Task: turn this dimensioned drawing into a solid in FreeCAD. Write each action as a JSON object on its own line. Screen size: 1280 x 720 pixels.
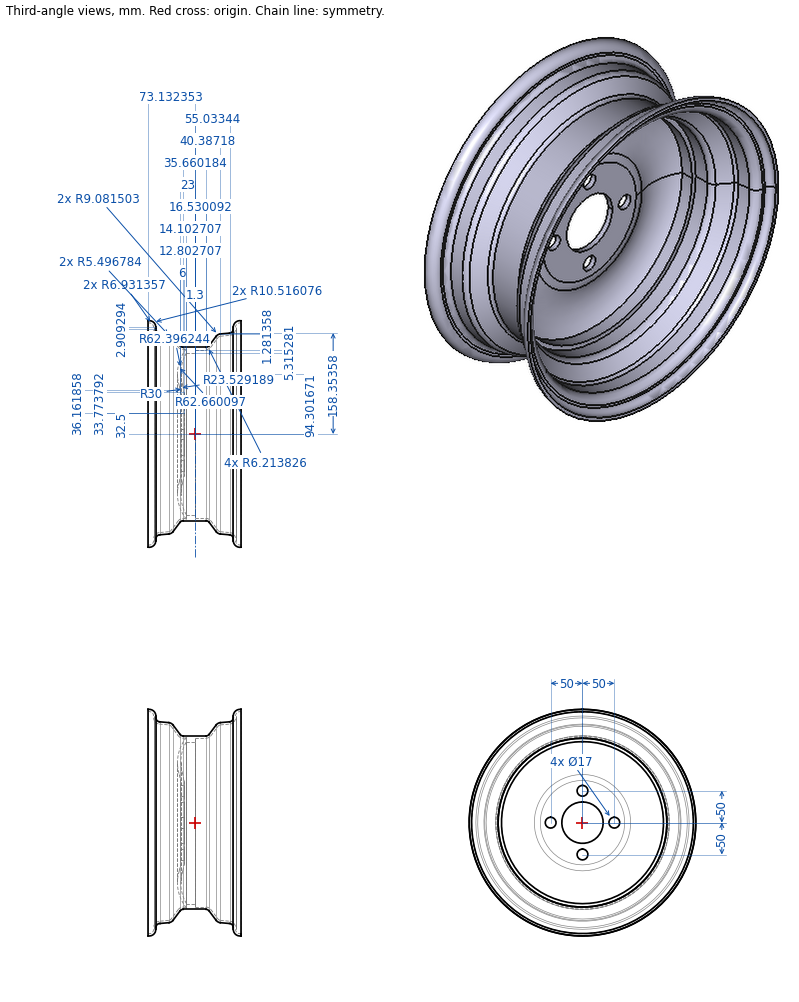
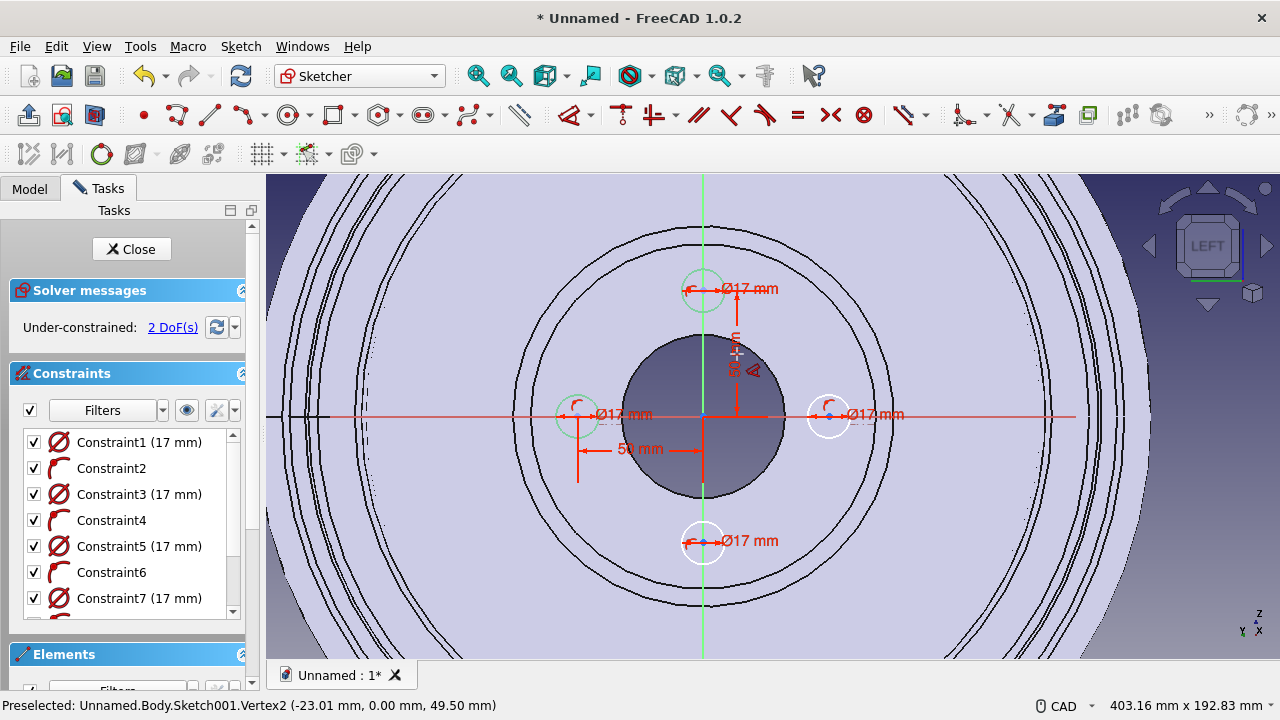
{"action": "left_click", "coordinate": [829, 416]}
{"action": "left_click", "coordinate": [766, 450]}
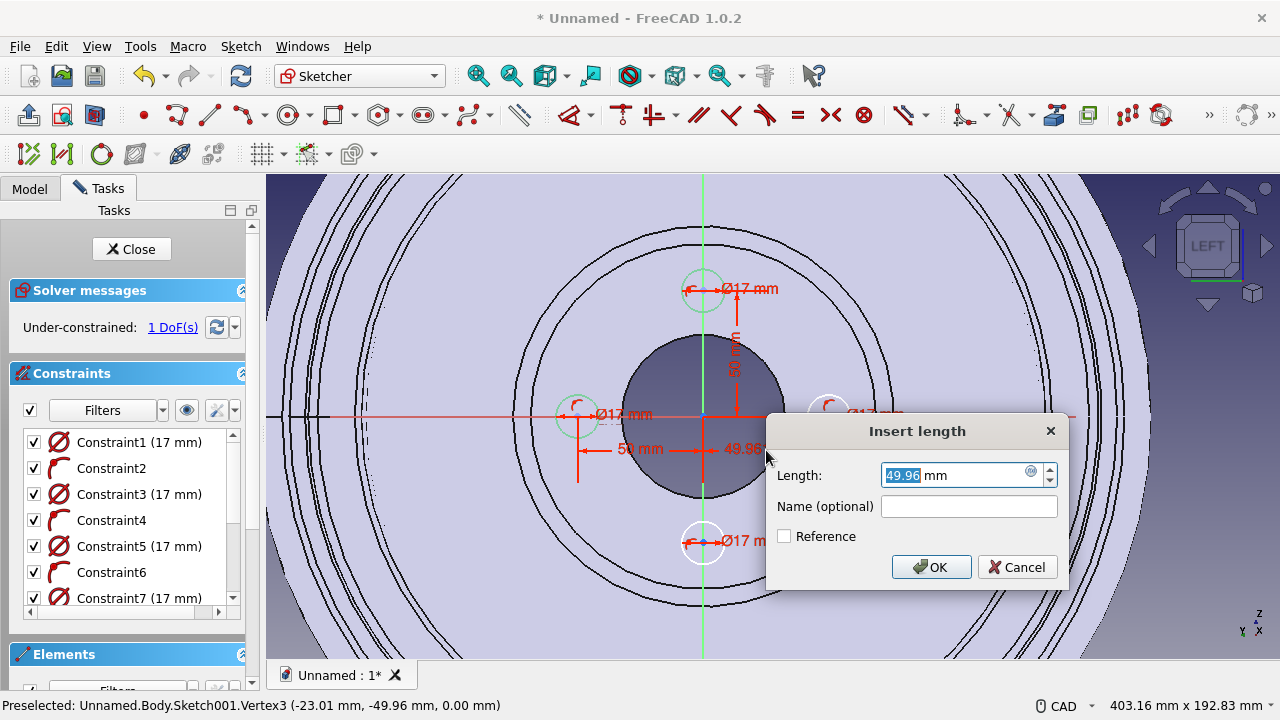
{"action": "type", "text": "50"}
{"action": "key", "text": "Return"}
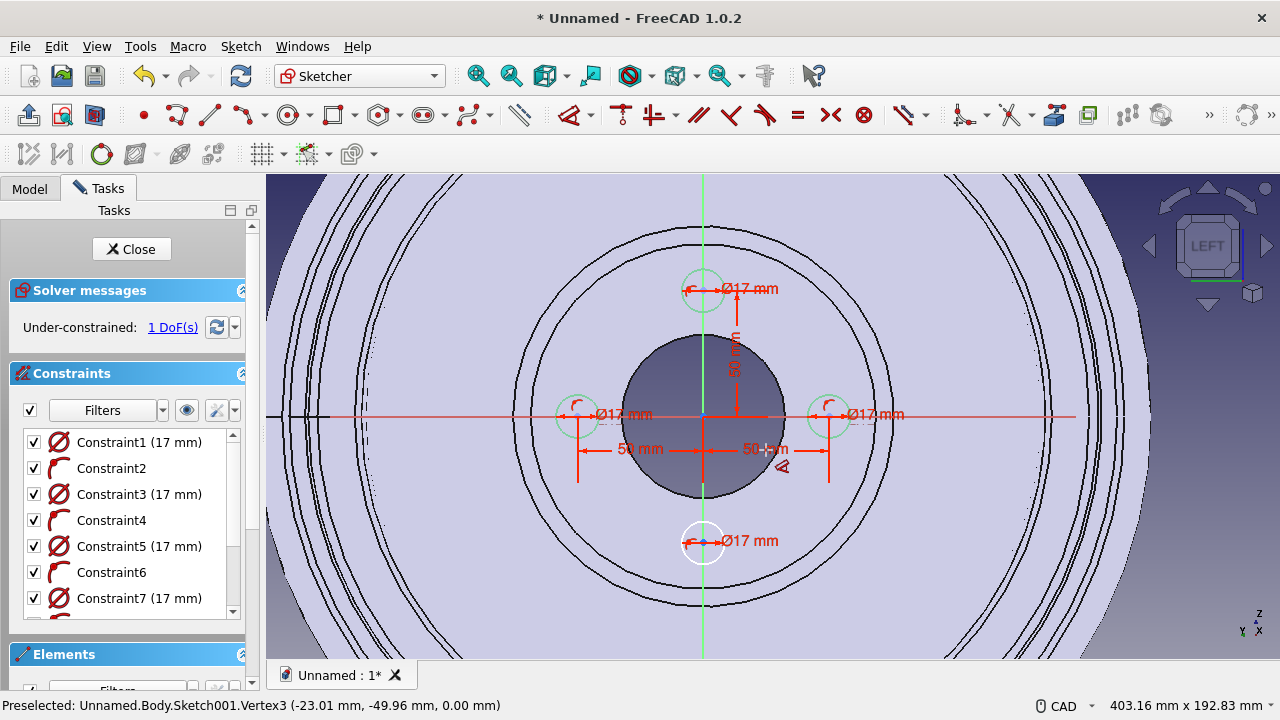
{"action": "left_click", "coordinate": [703, 543]}
{"action": "left_click", "coordinate": [737, 480]}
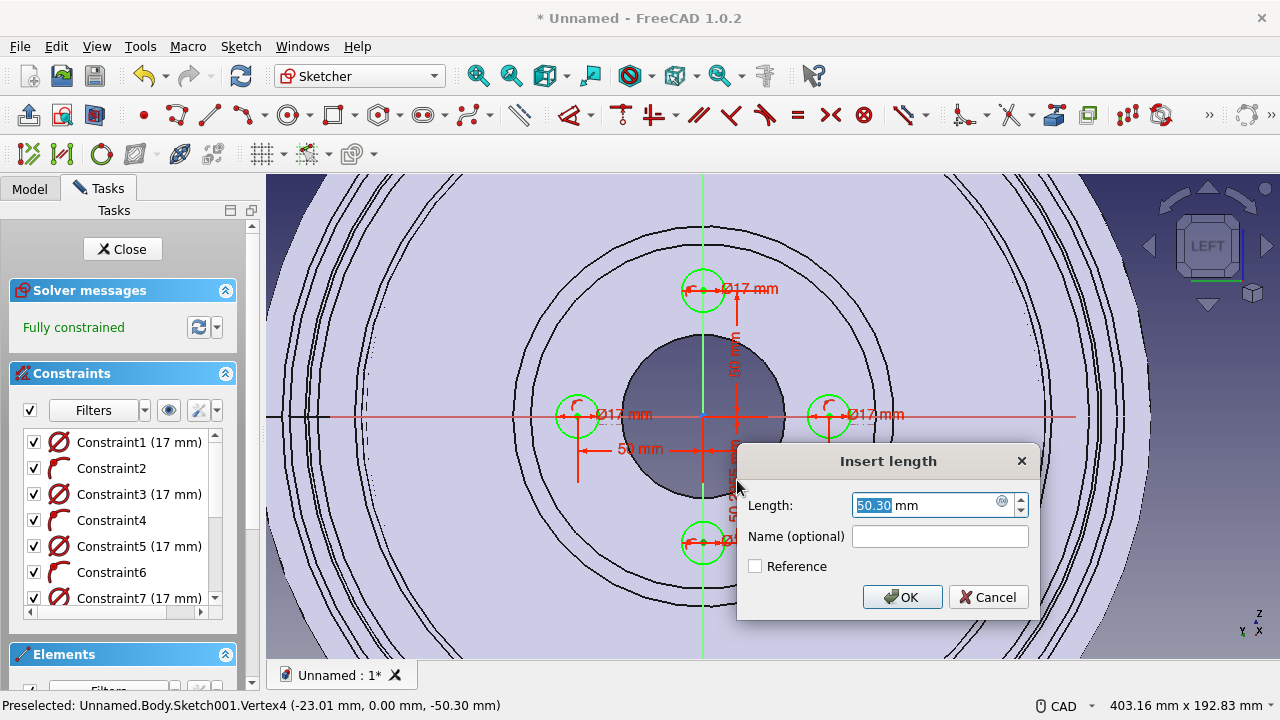
{"action": "type", "text": "50"}
{"action": "key", "text": "Return"}
{"action": "key", "text": "Escape"}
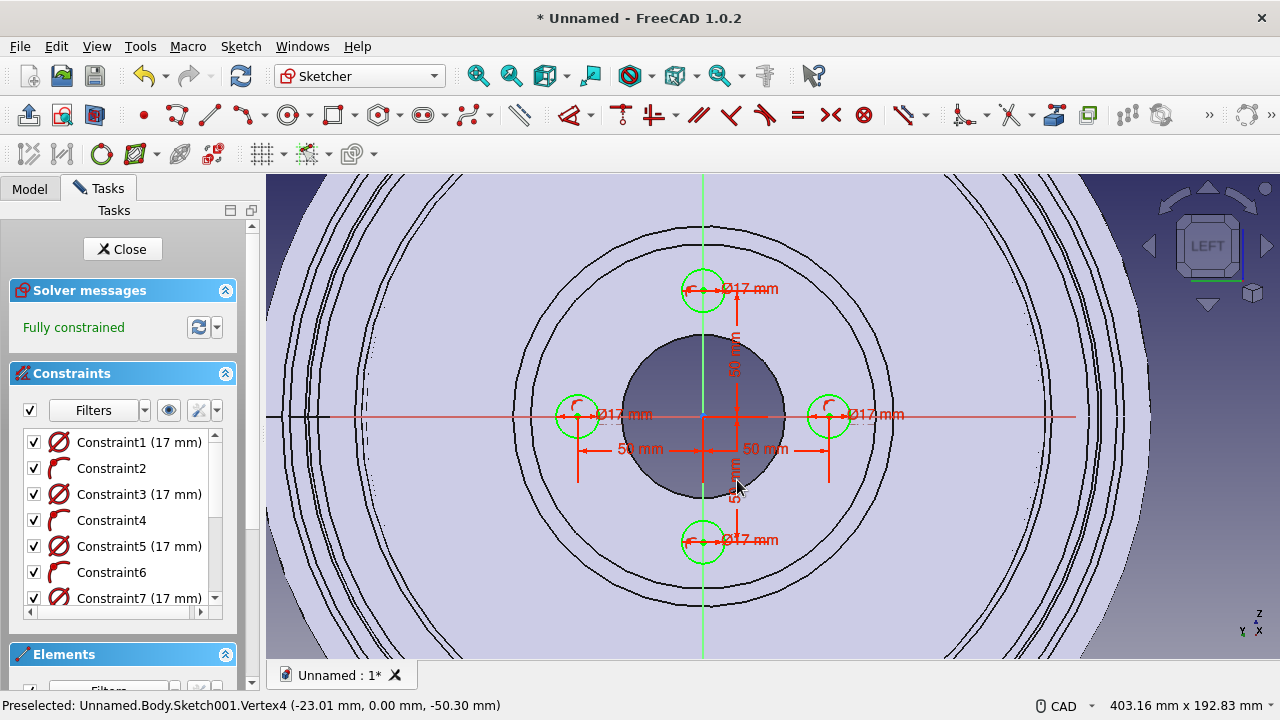
{"action": "left_click", "coordinate": [123, 249]}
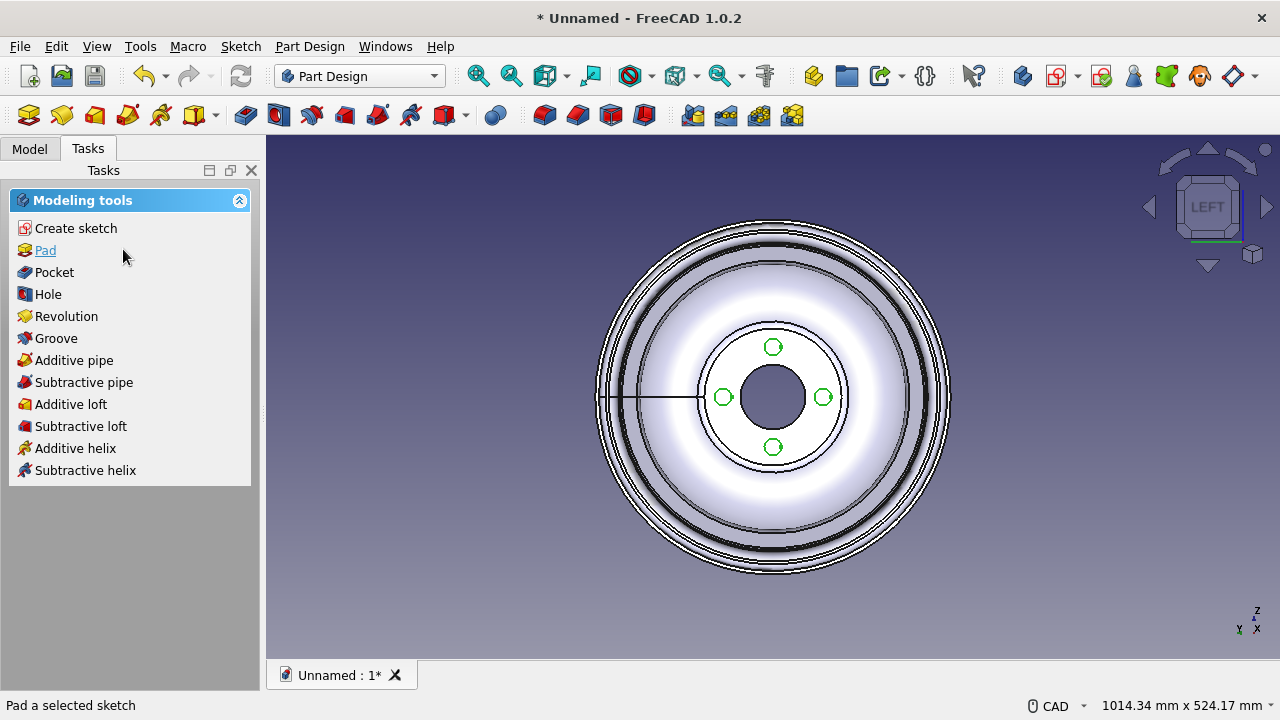
{"action": "left_click", "coordinate": [246, 116]}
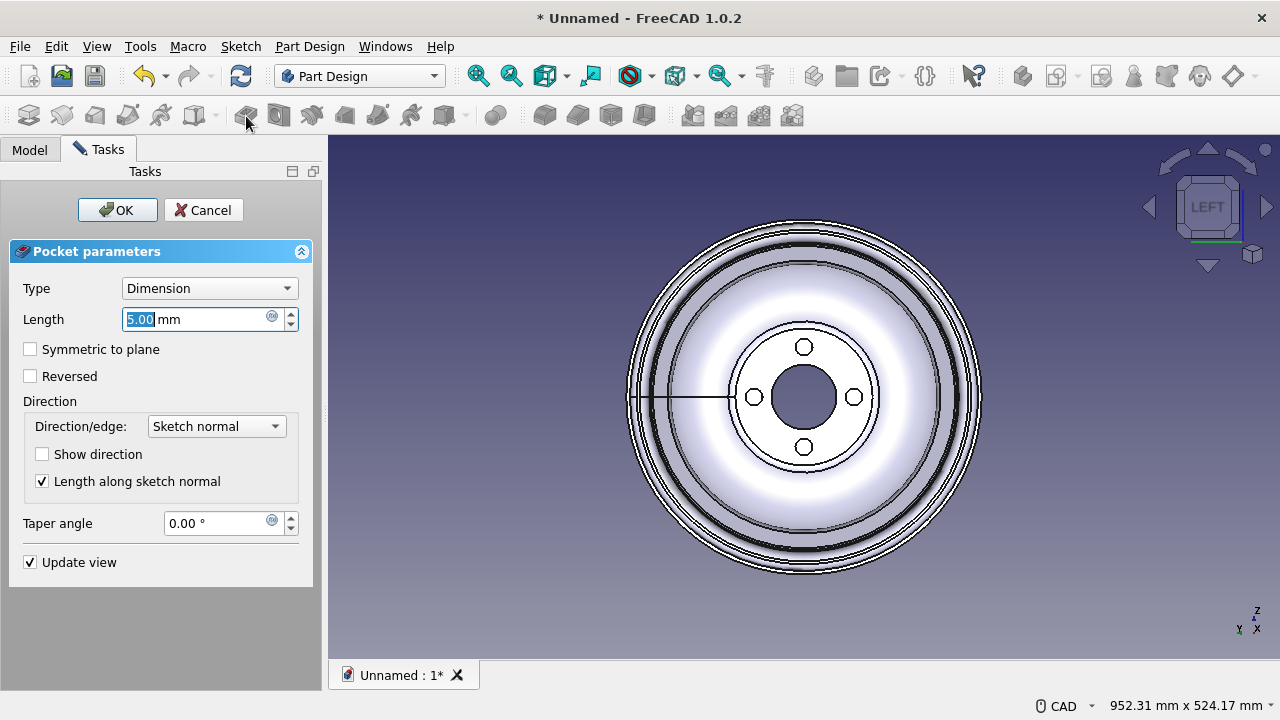
{"action": "left_click", "coordinate": [210, 288]}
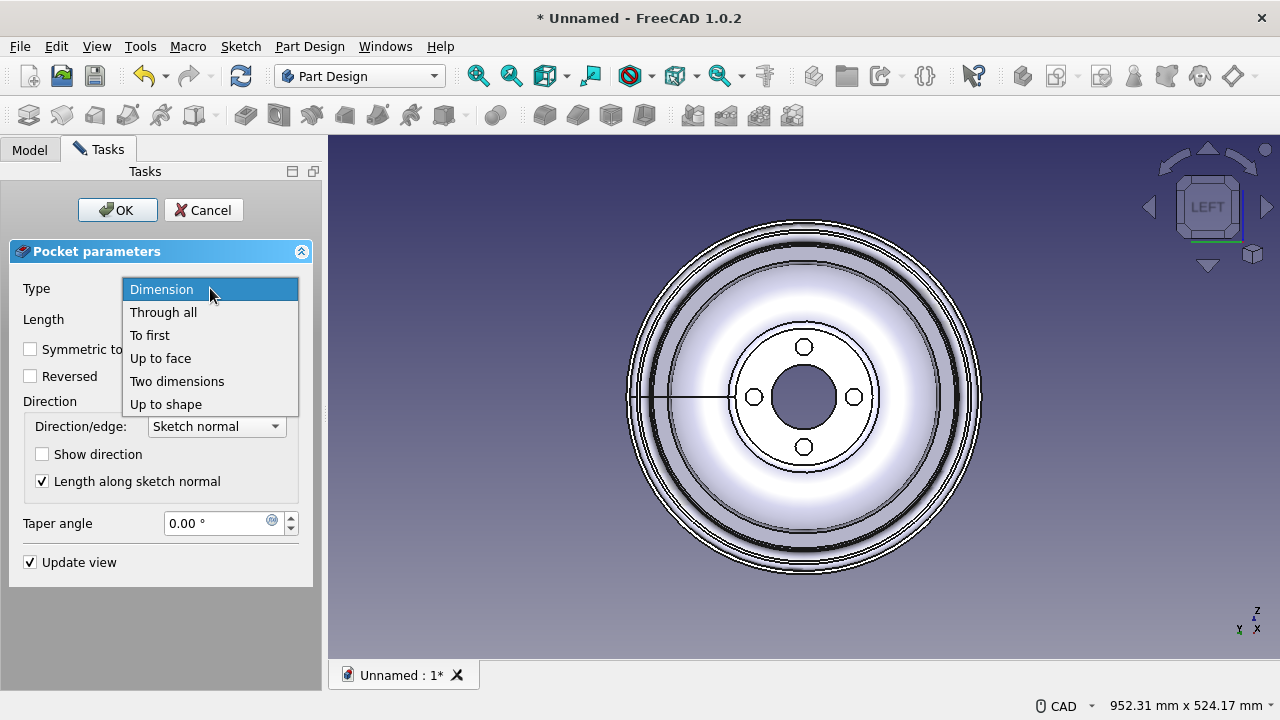
{"action": "left_click", "coordinate": [208, 312]}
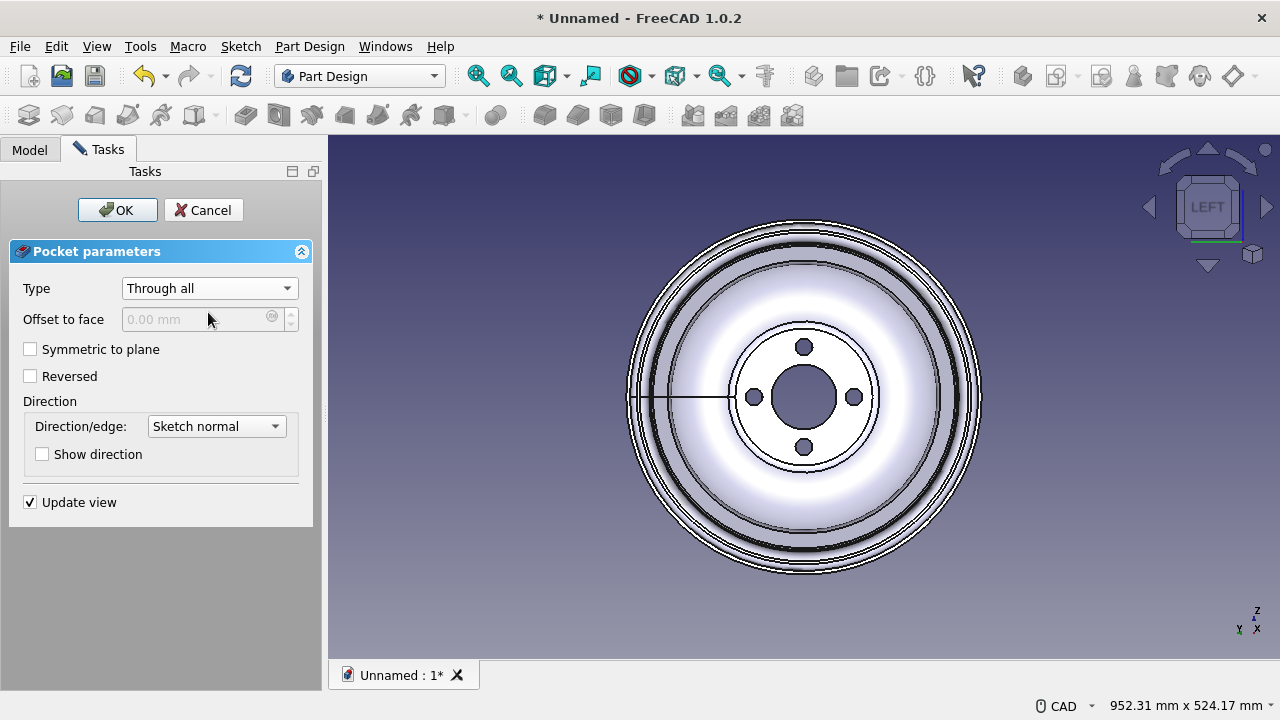
{"action": "left_click", "coordinate": [118, 210]}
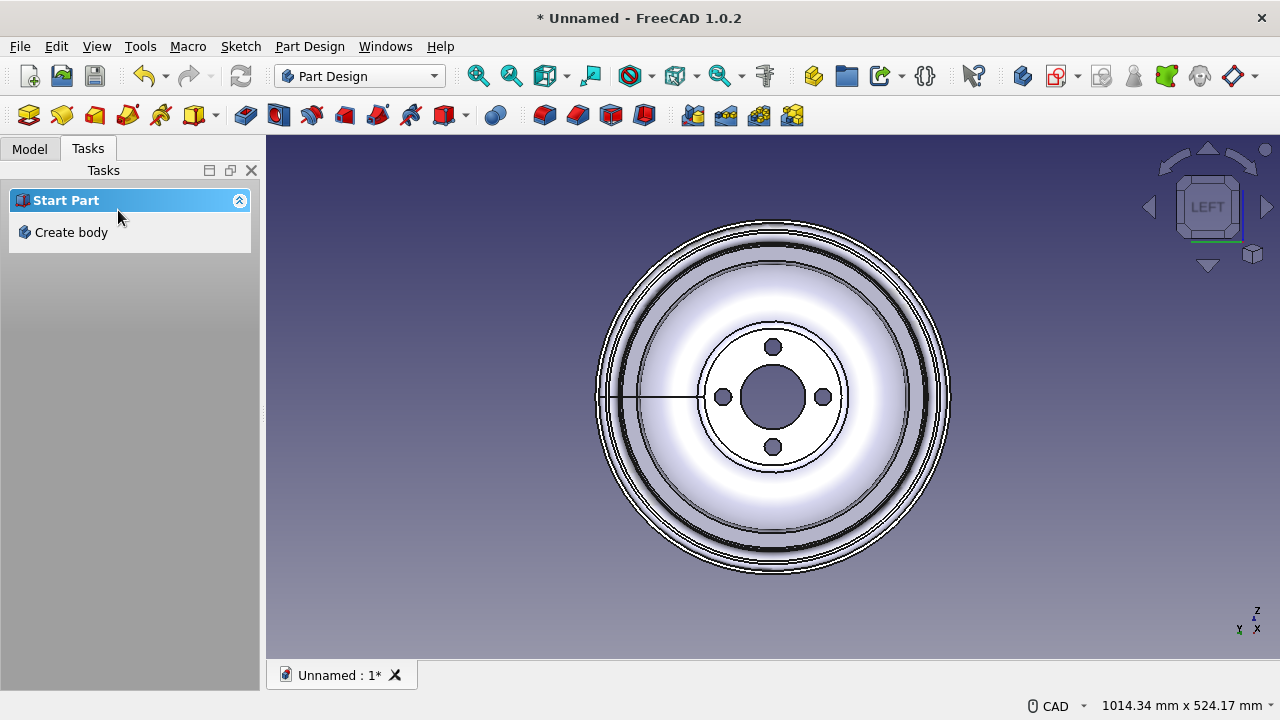
{"action": "key", "text": "0"}